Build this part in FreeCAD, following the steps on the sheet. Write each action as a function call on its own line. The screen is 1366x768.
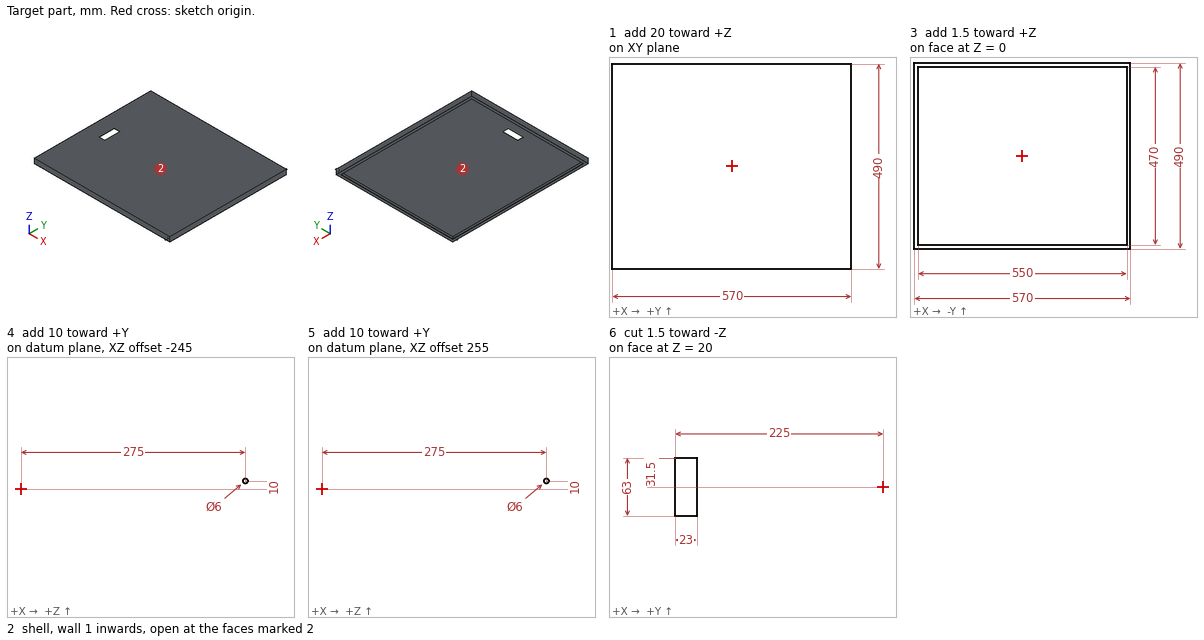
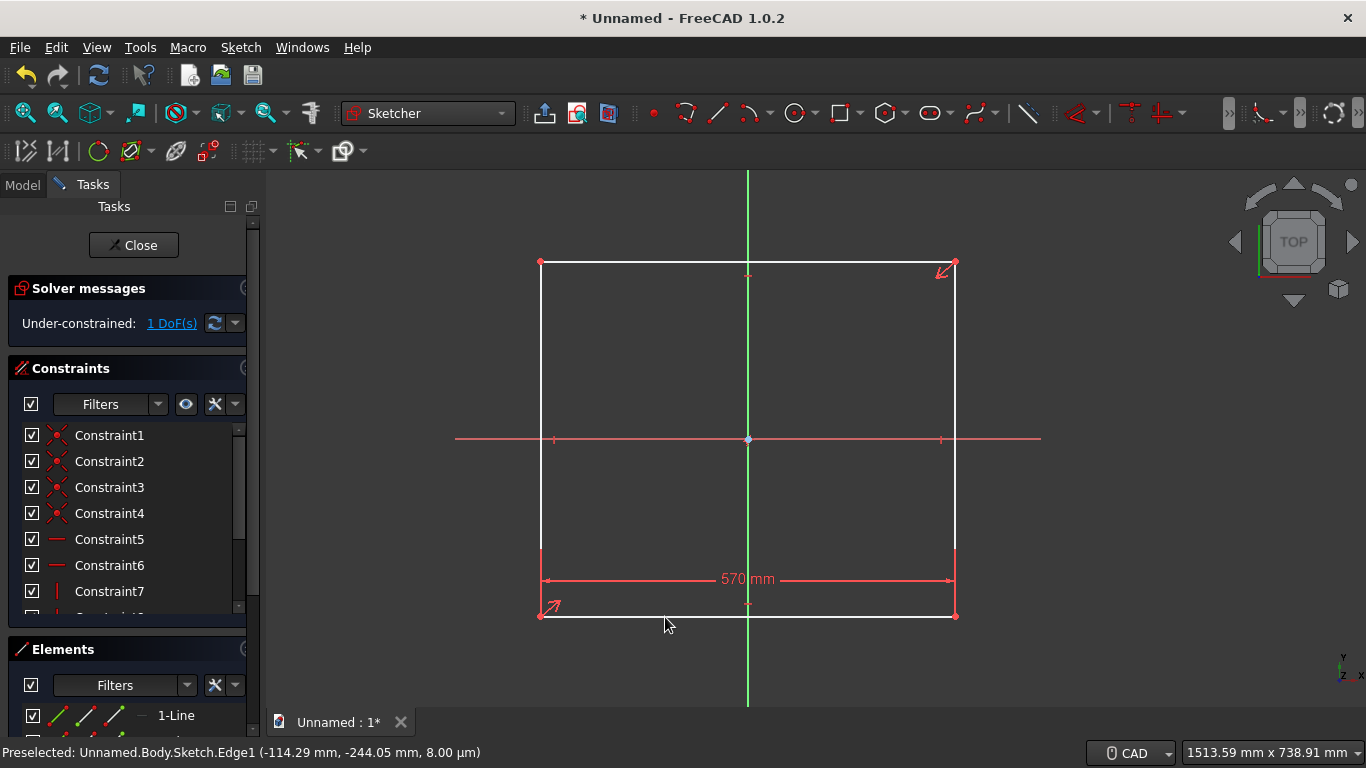
click(955, 510)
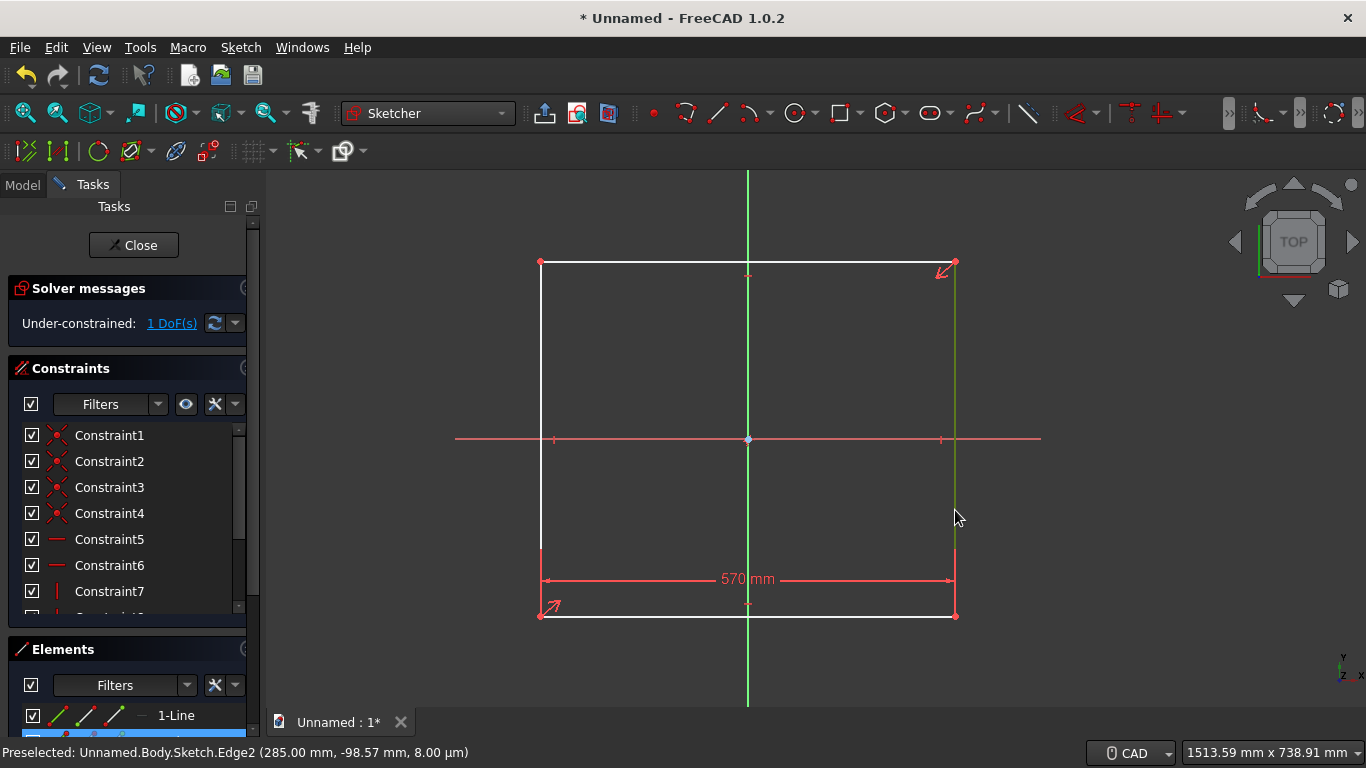
key(i)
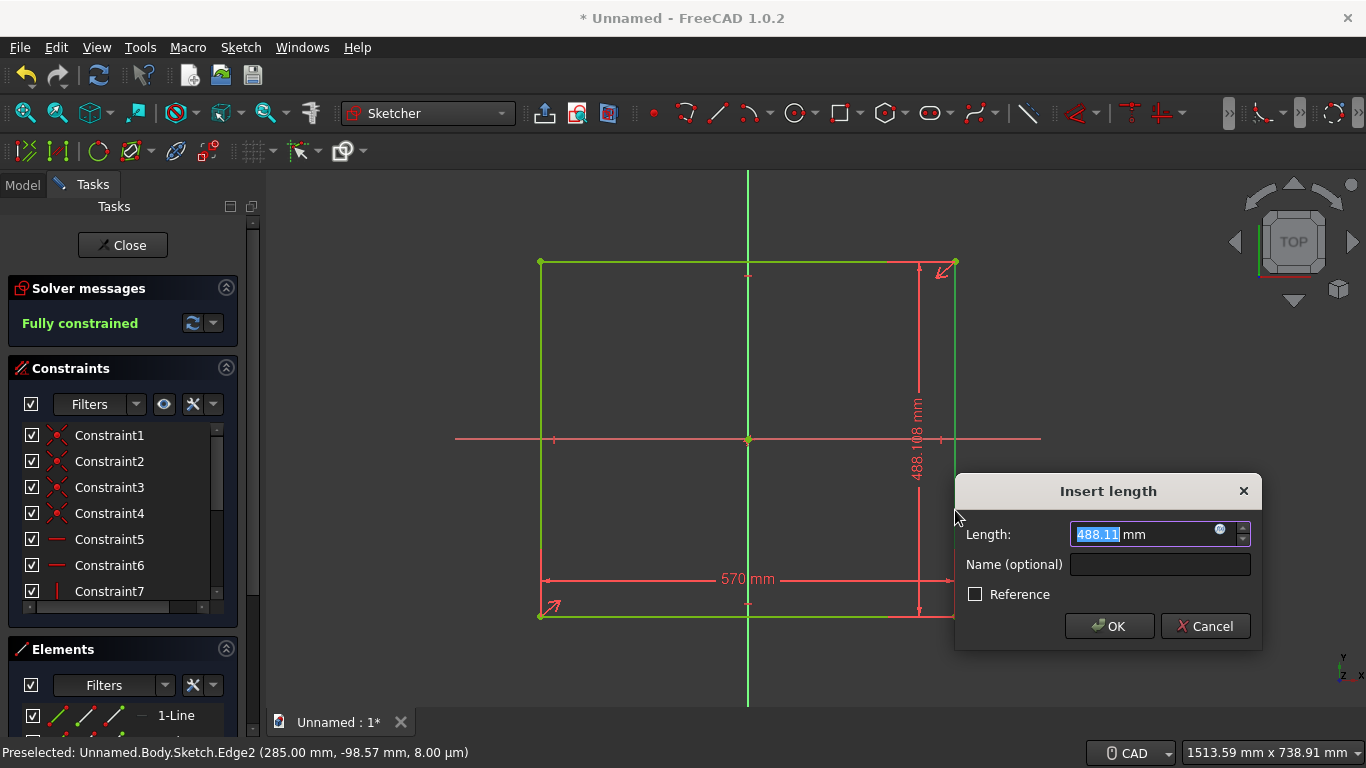
text(490)
key(Return)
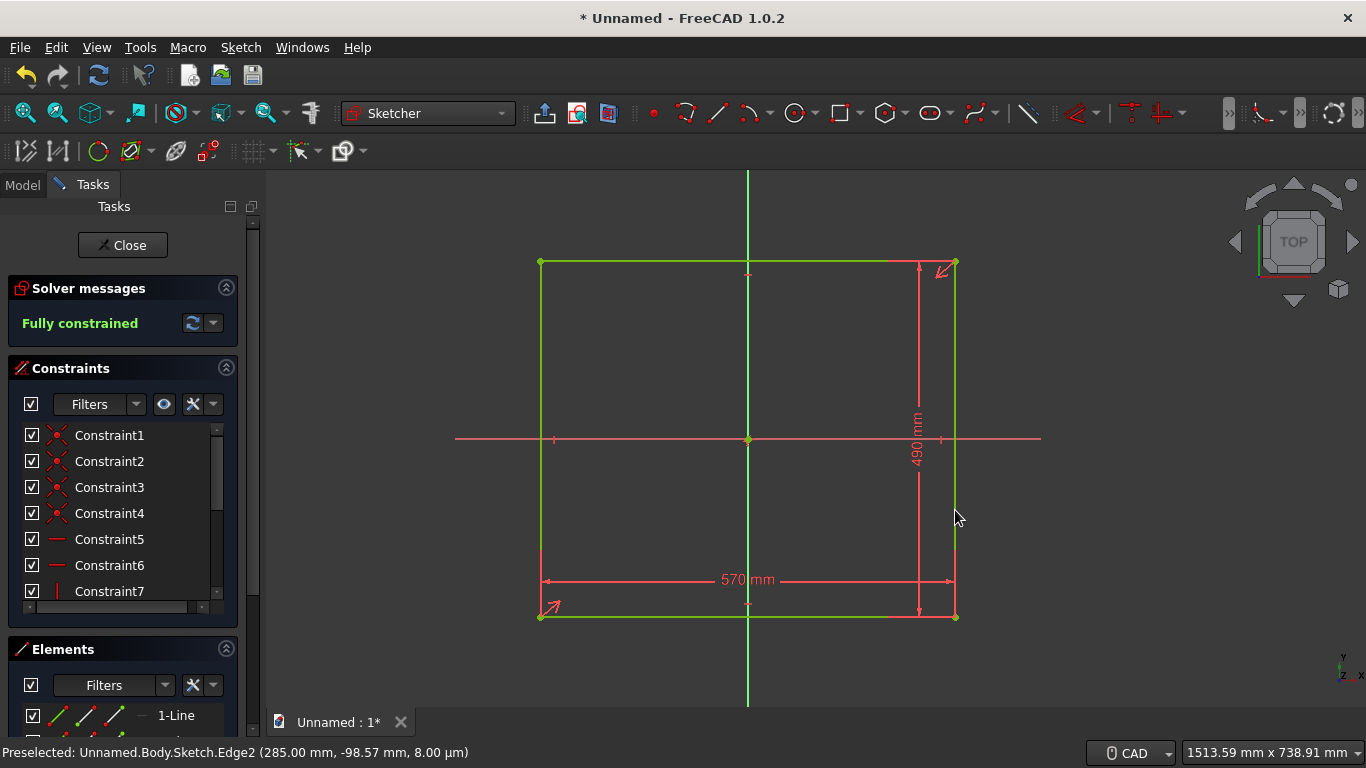
click(123, 245)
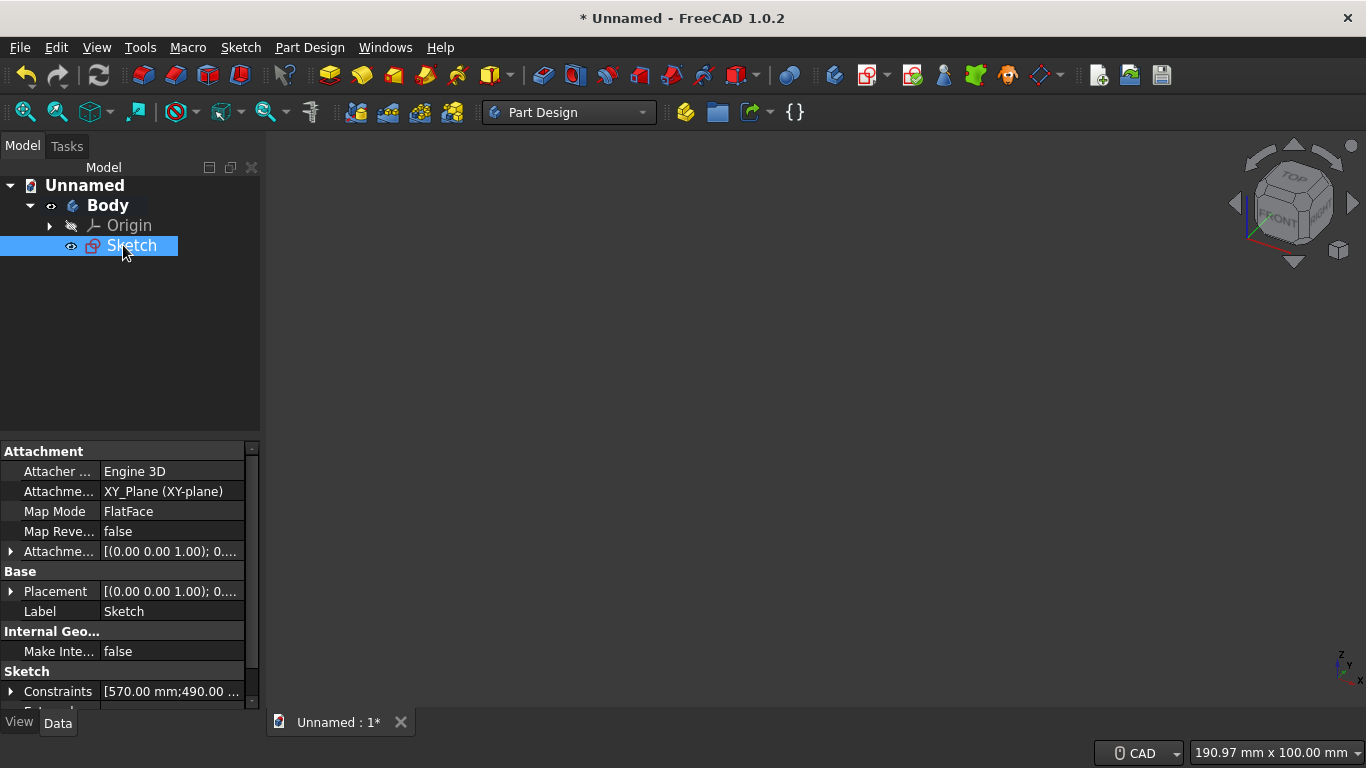
click(330, 76)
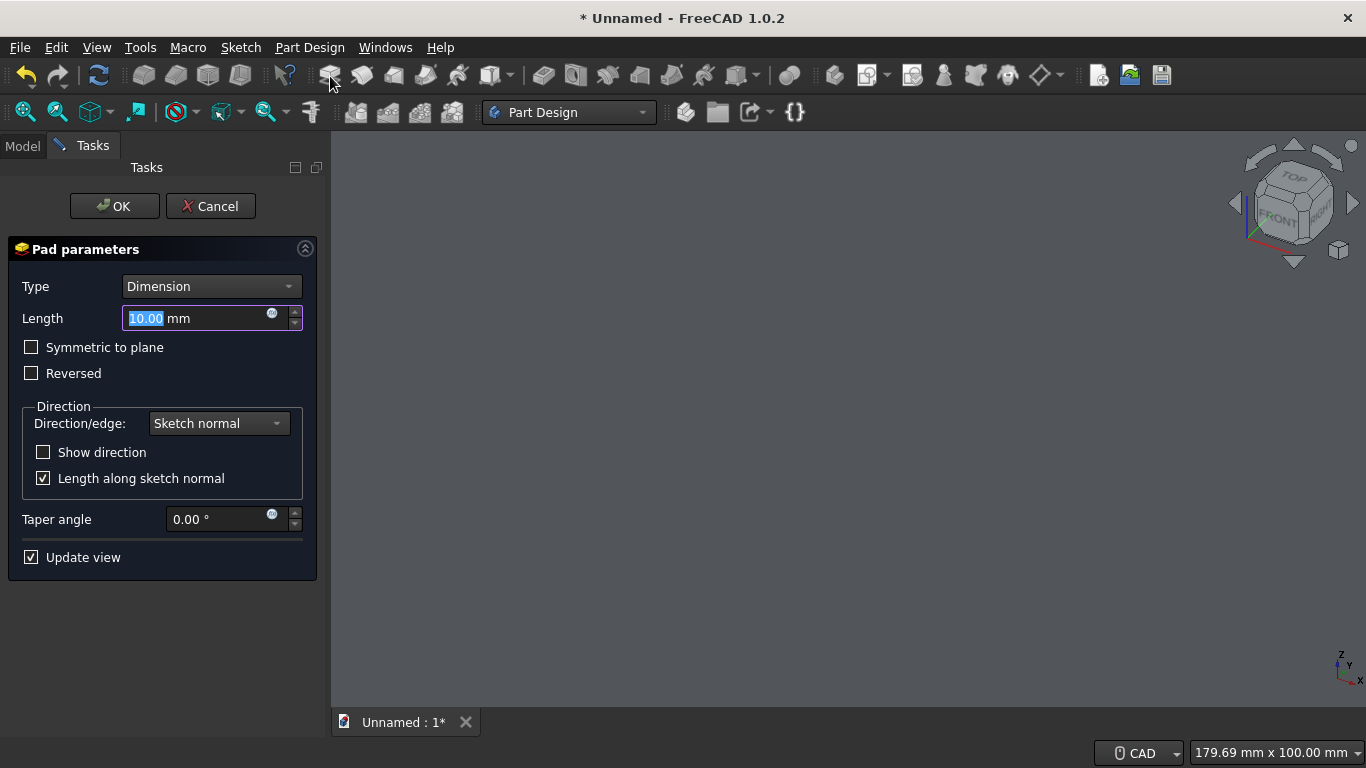
text(20)
key(Tab)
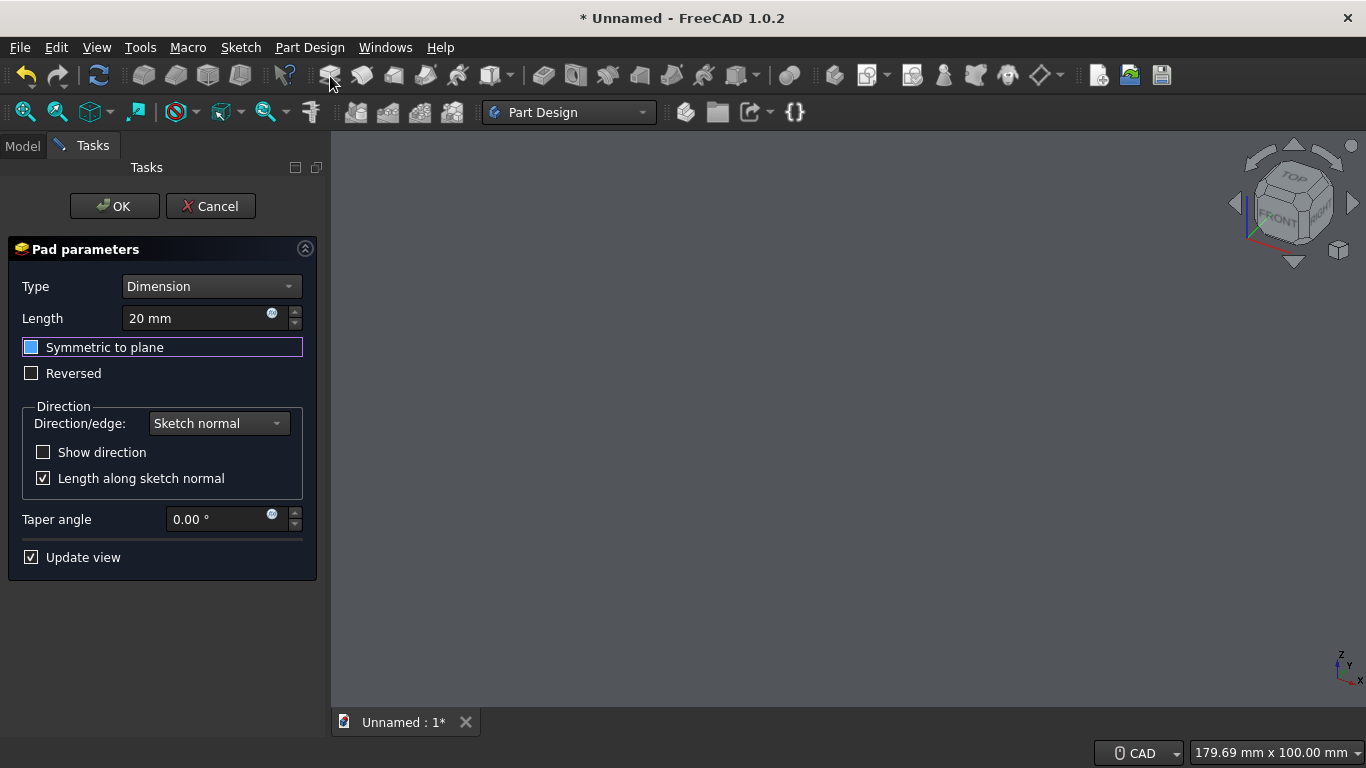
click(115, 206)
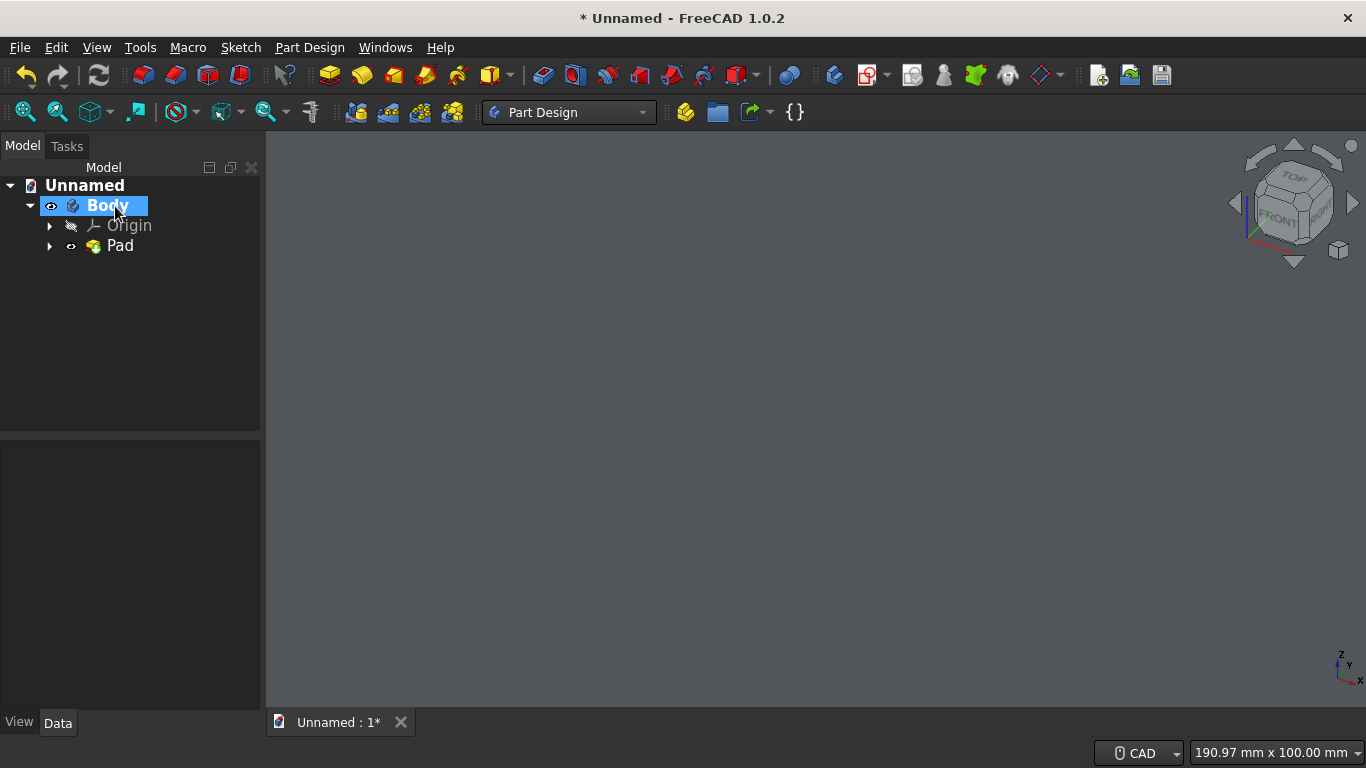
key(v)
key(f)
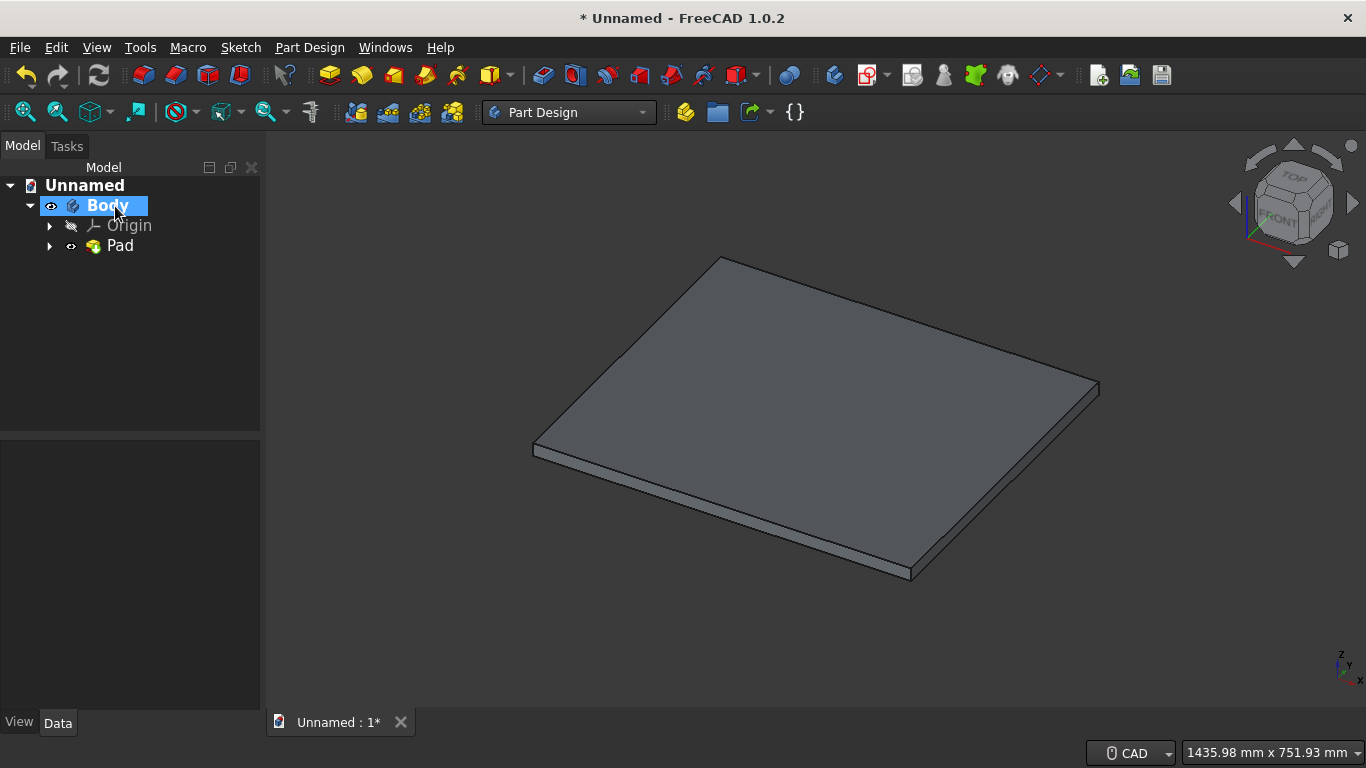
key(0)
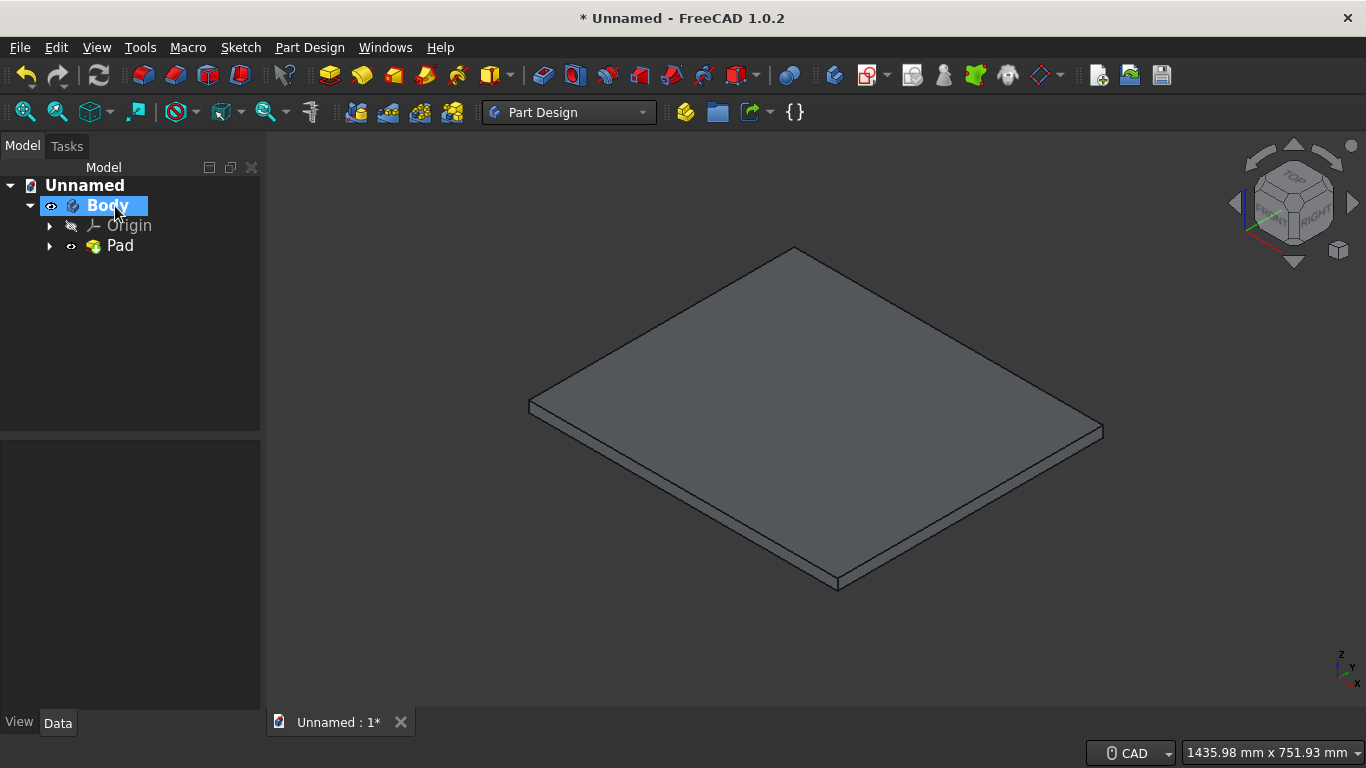
key(2)